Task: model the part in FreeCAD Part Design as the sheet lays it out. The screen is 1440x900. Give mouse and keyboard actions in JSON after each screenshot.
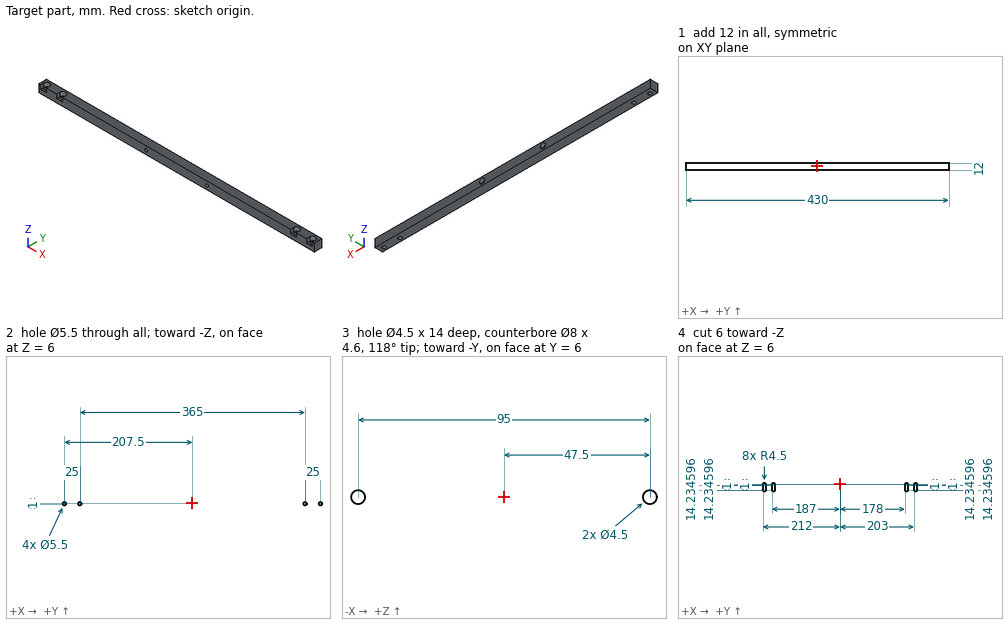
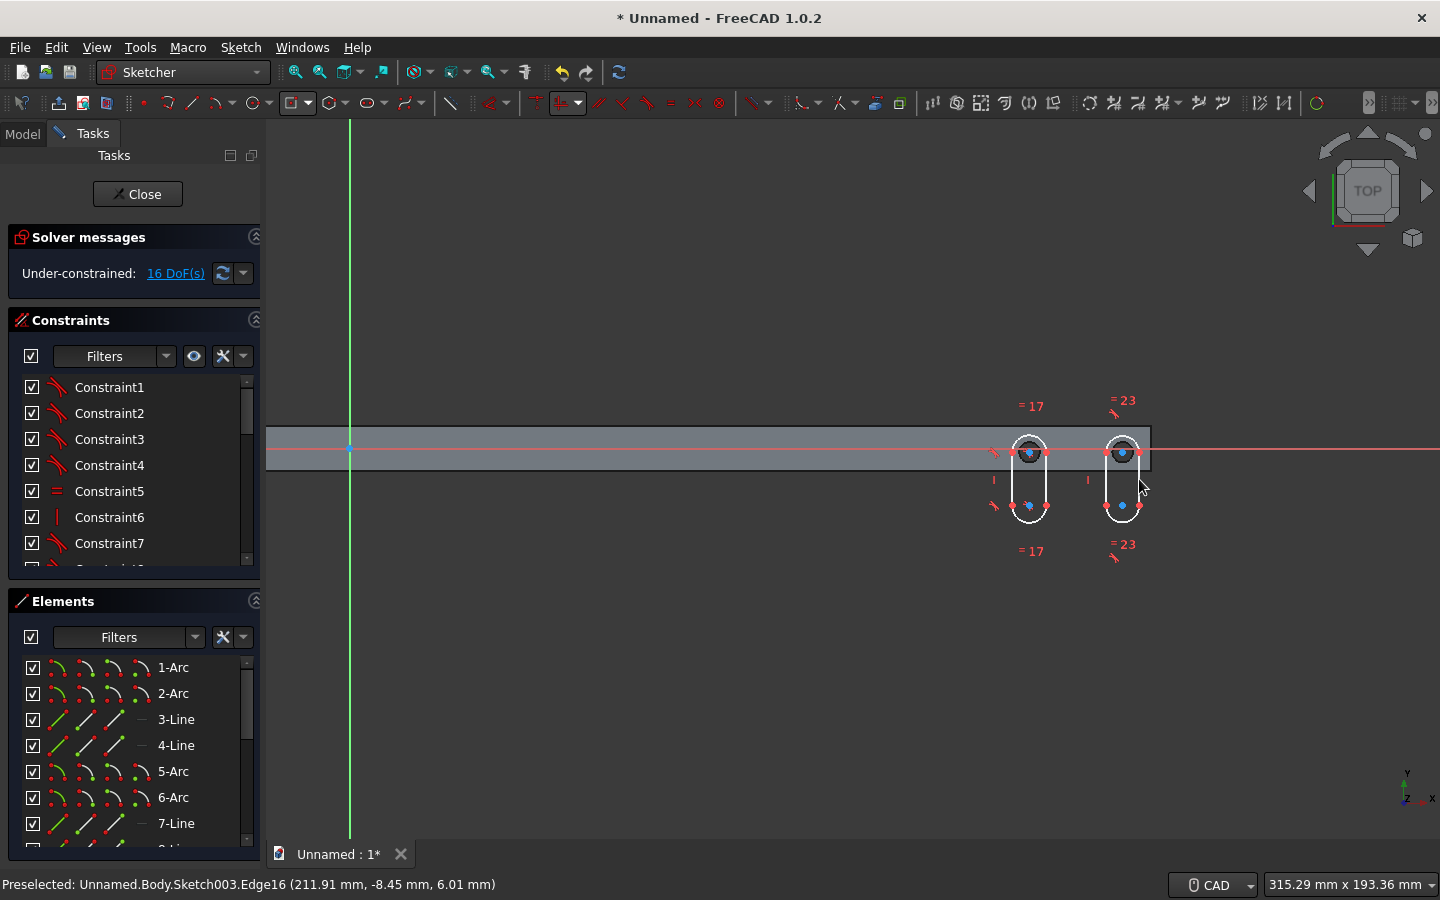
{"action": "scroll", "coordinate": [1139, 479], "scroll_direction": "down", "scroll_amount": 4}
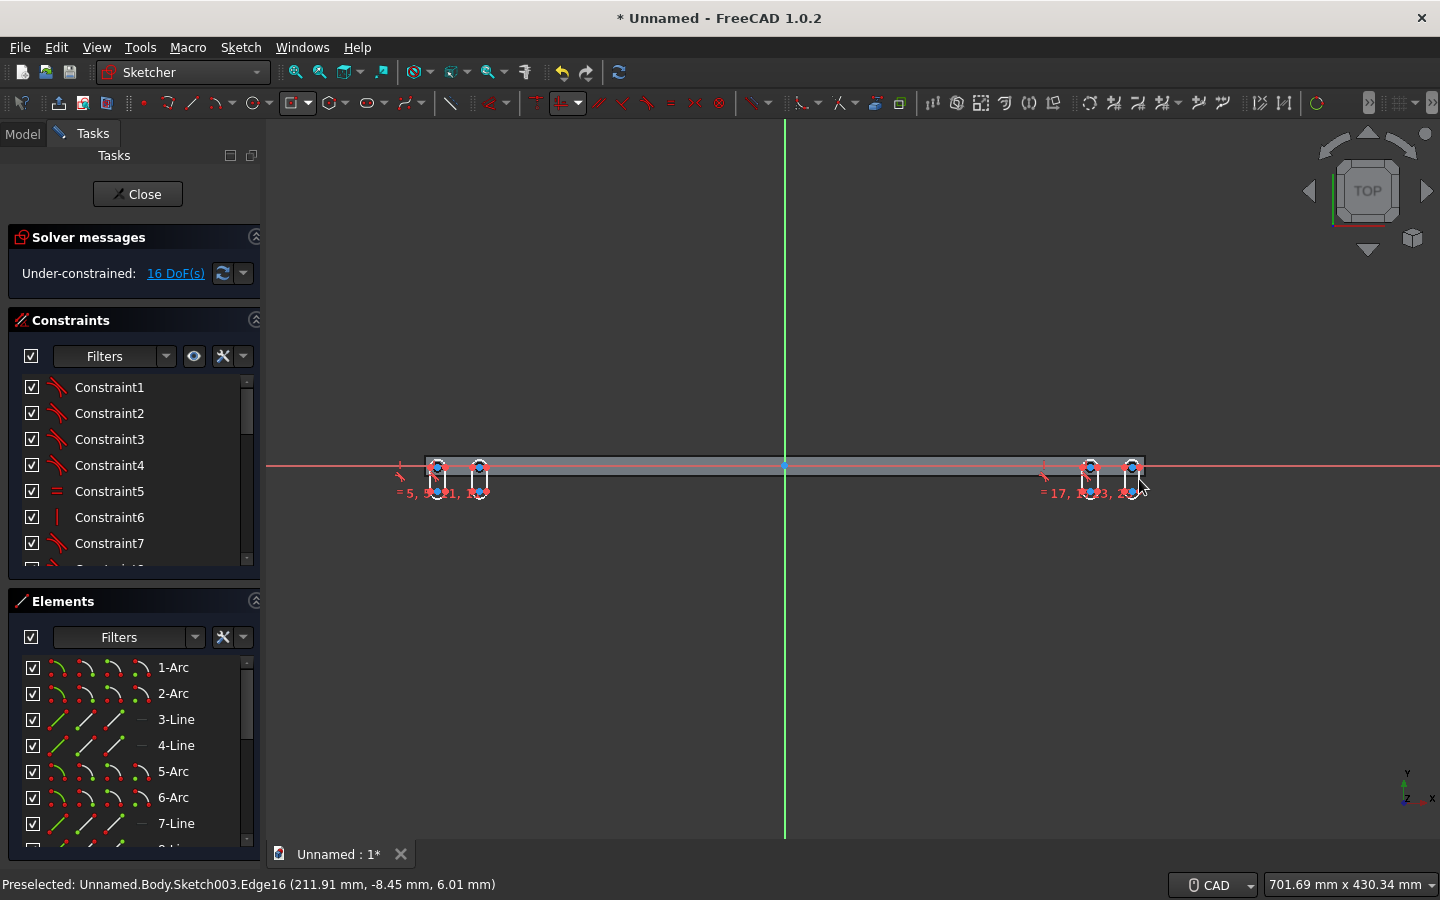
{"action": "scroll", "coordinate": [433, 497], "scroll_direction": "up", "scroll_amount": 4}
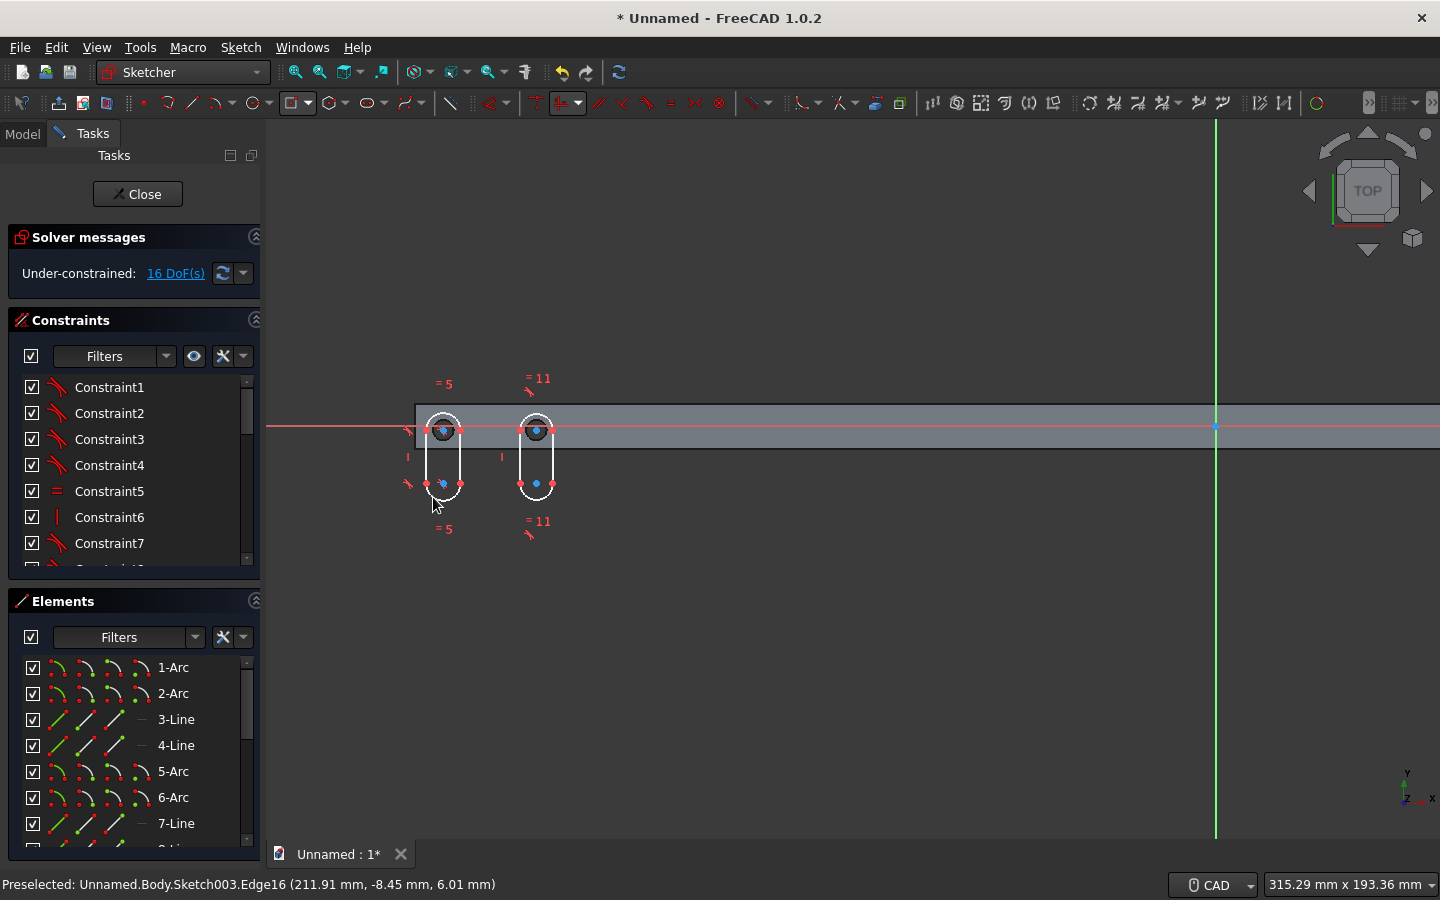
{"action": "left_click", "coordinate": [433, 497]}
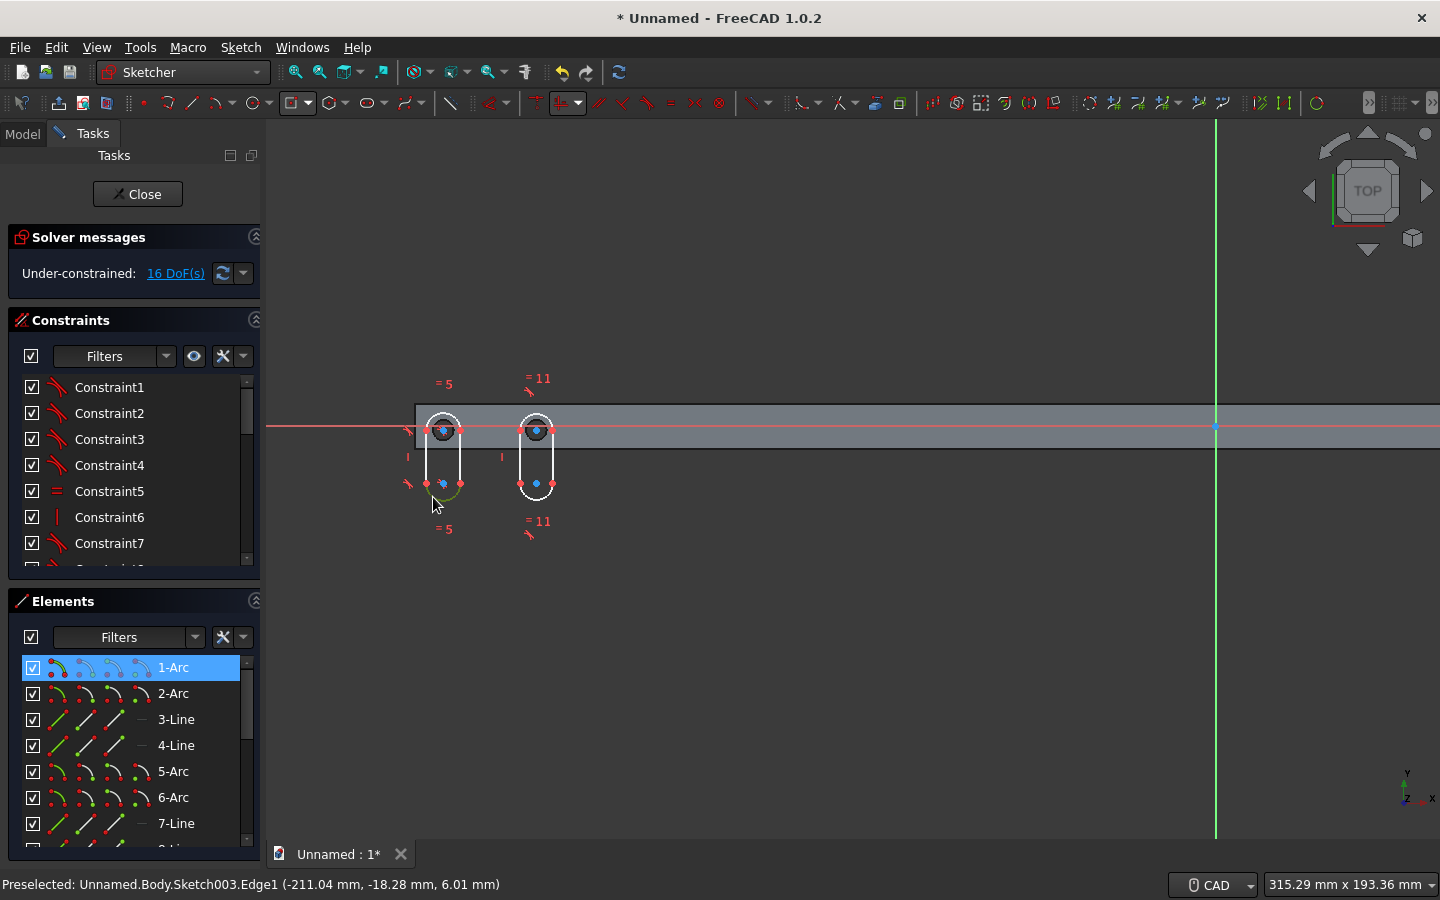
{"action": "left_click", "coordinate": [527, 497]}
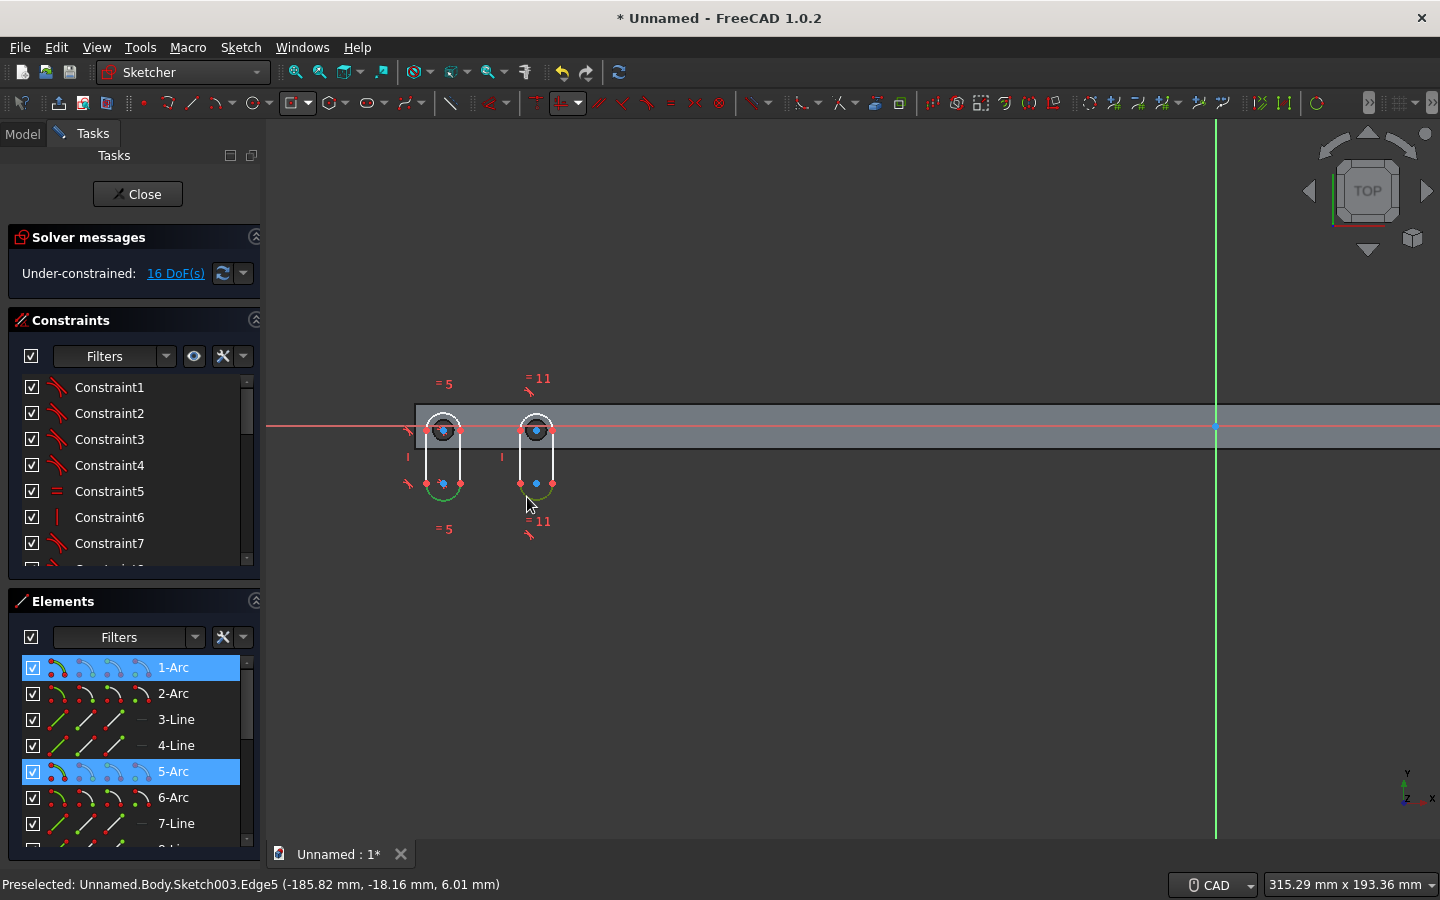
{"action": "scroll", "coordinate": [432, 497], "scroll_direction": "down", "scroll_amount": 4}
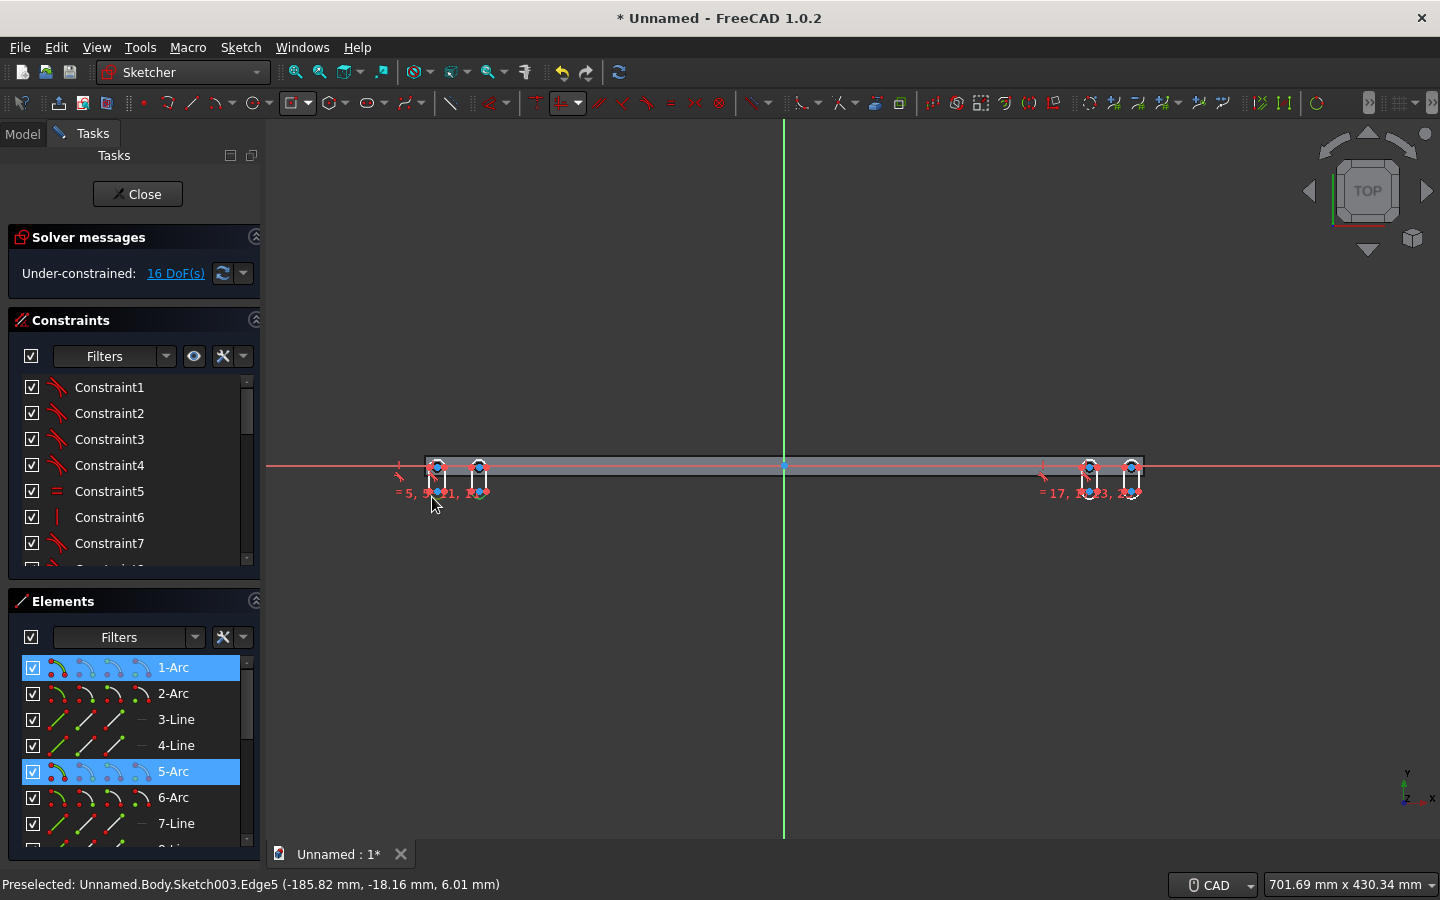
{"action": "scroll", "coordinate": [1085, 497], "scroll_direction": "up", "scroll_amount": 4}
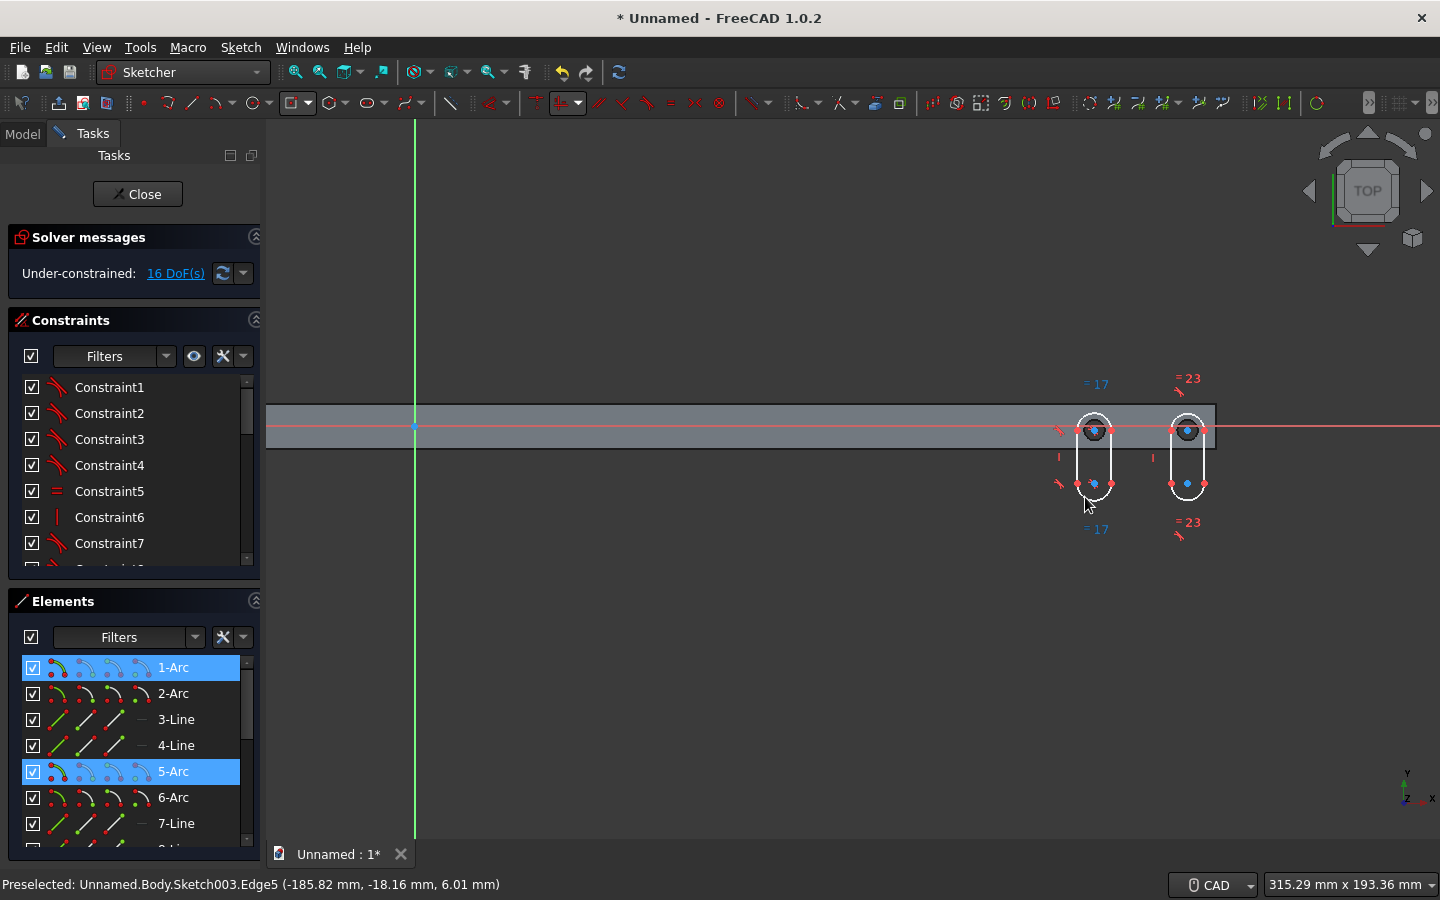
{"action": "left_click", "coordinate": [1084, 497]}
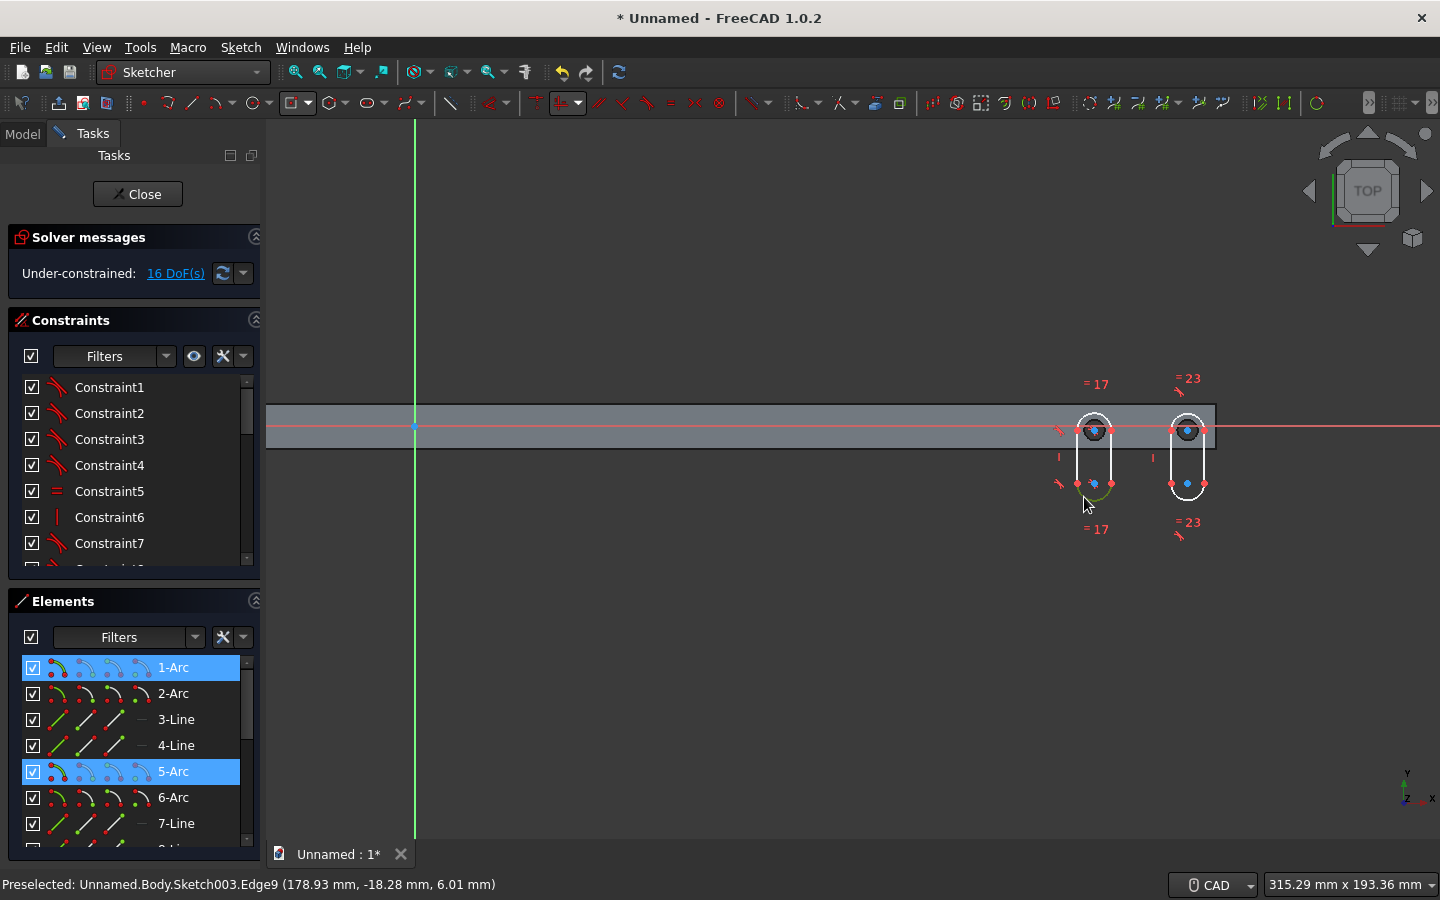
{"action": "left_click", "coordinate": [1178, 497]}